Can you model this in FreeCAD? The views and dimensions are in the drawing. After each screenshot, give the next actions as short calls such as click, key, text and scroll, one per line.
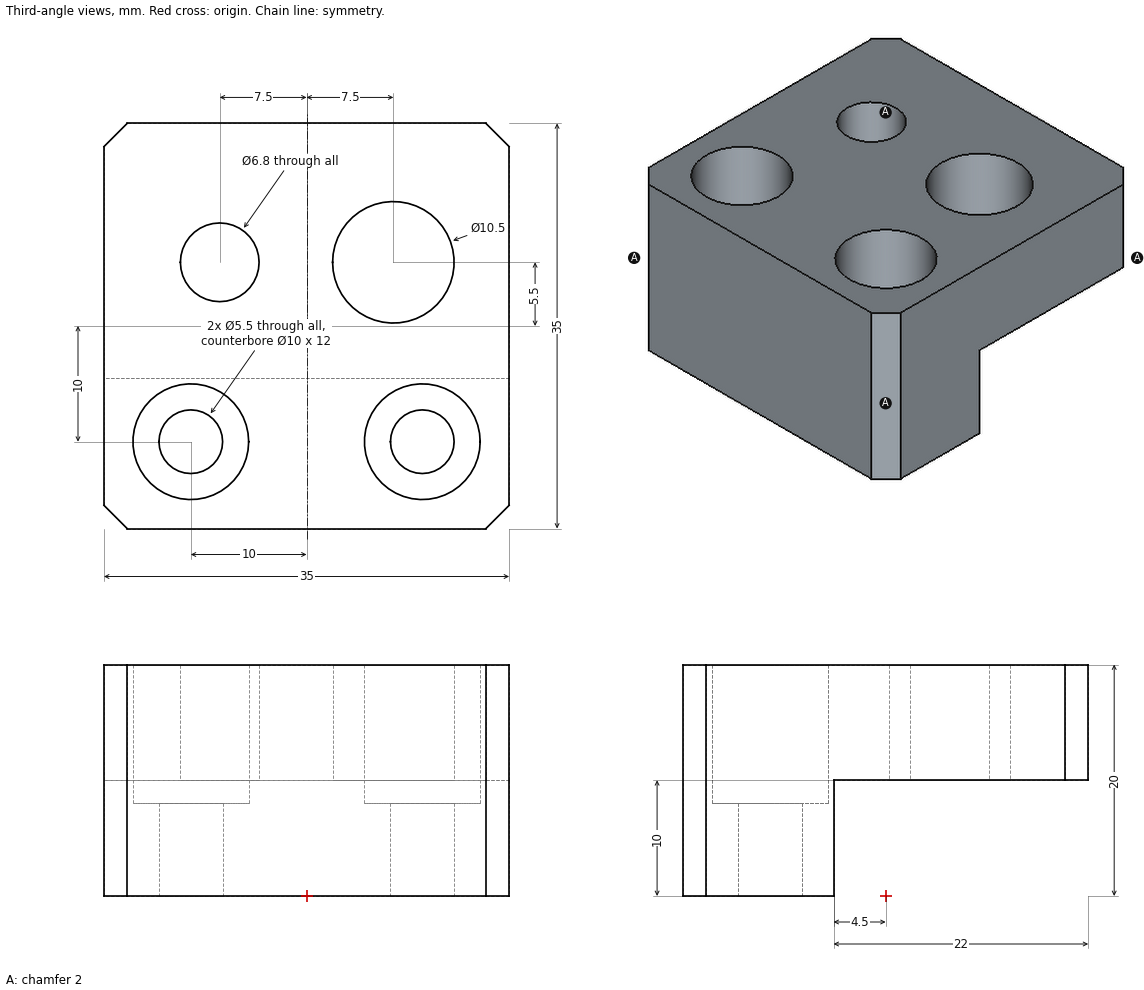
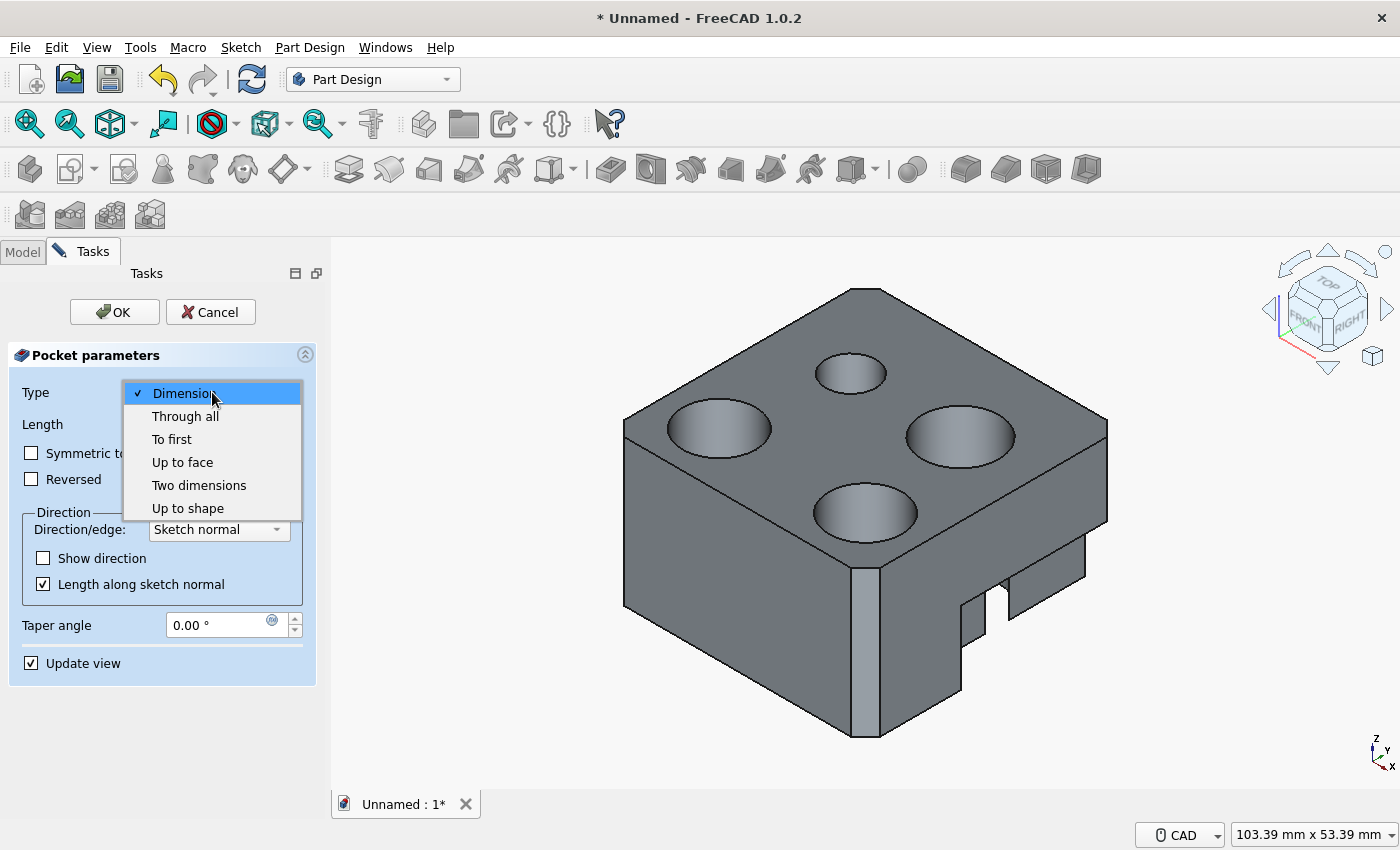
click(212, 416)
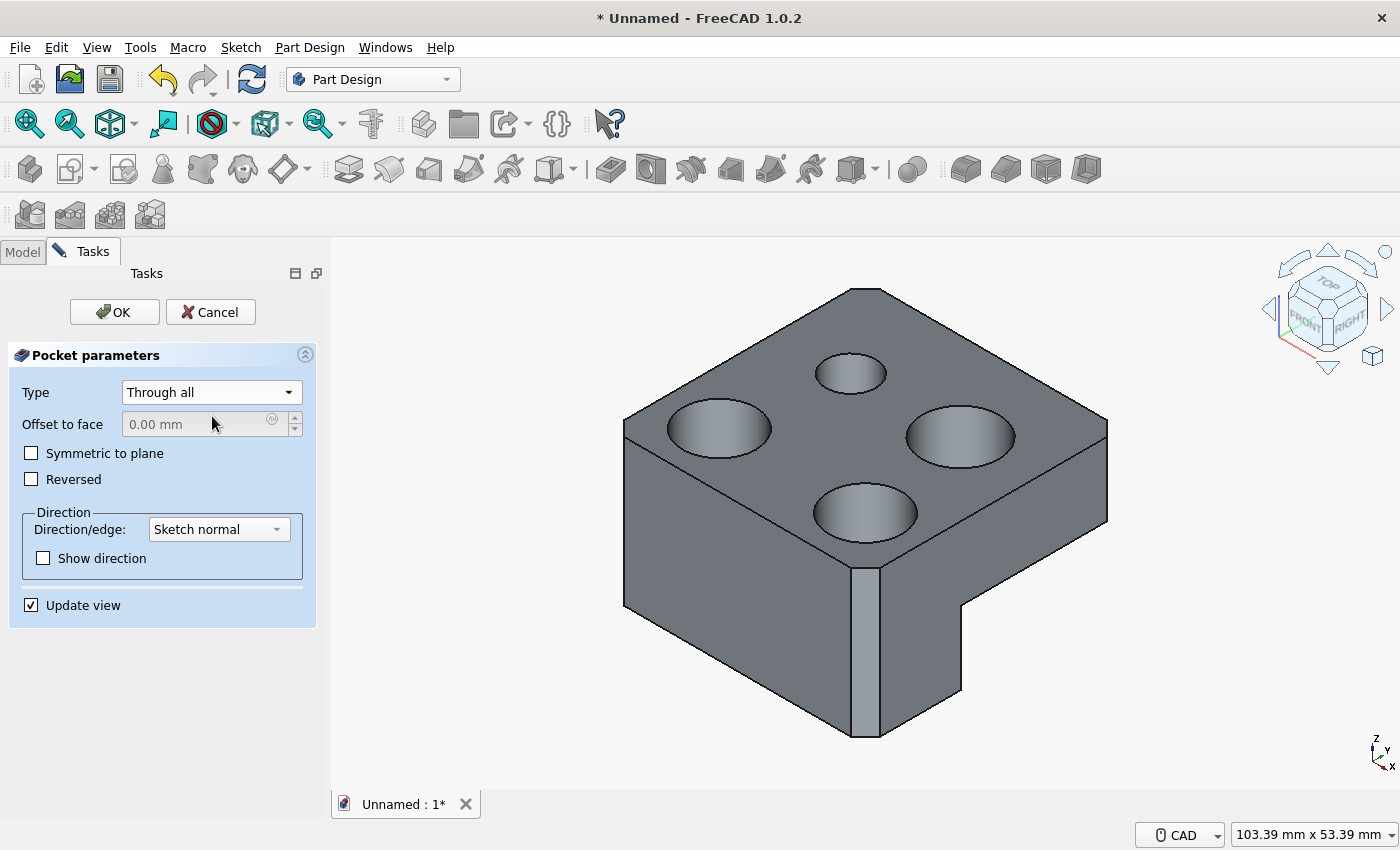
click(115, 312)